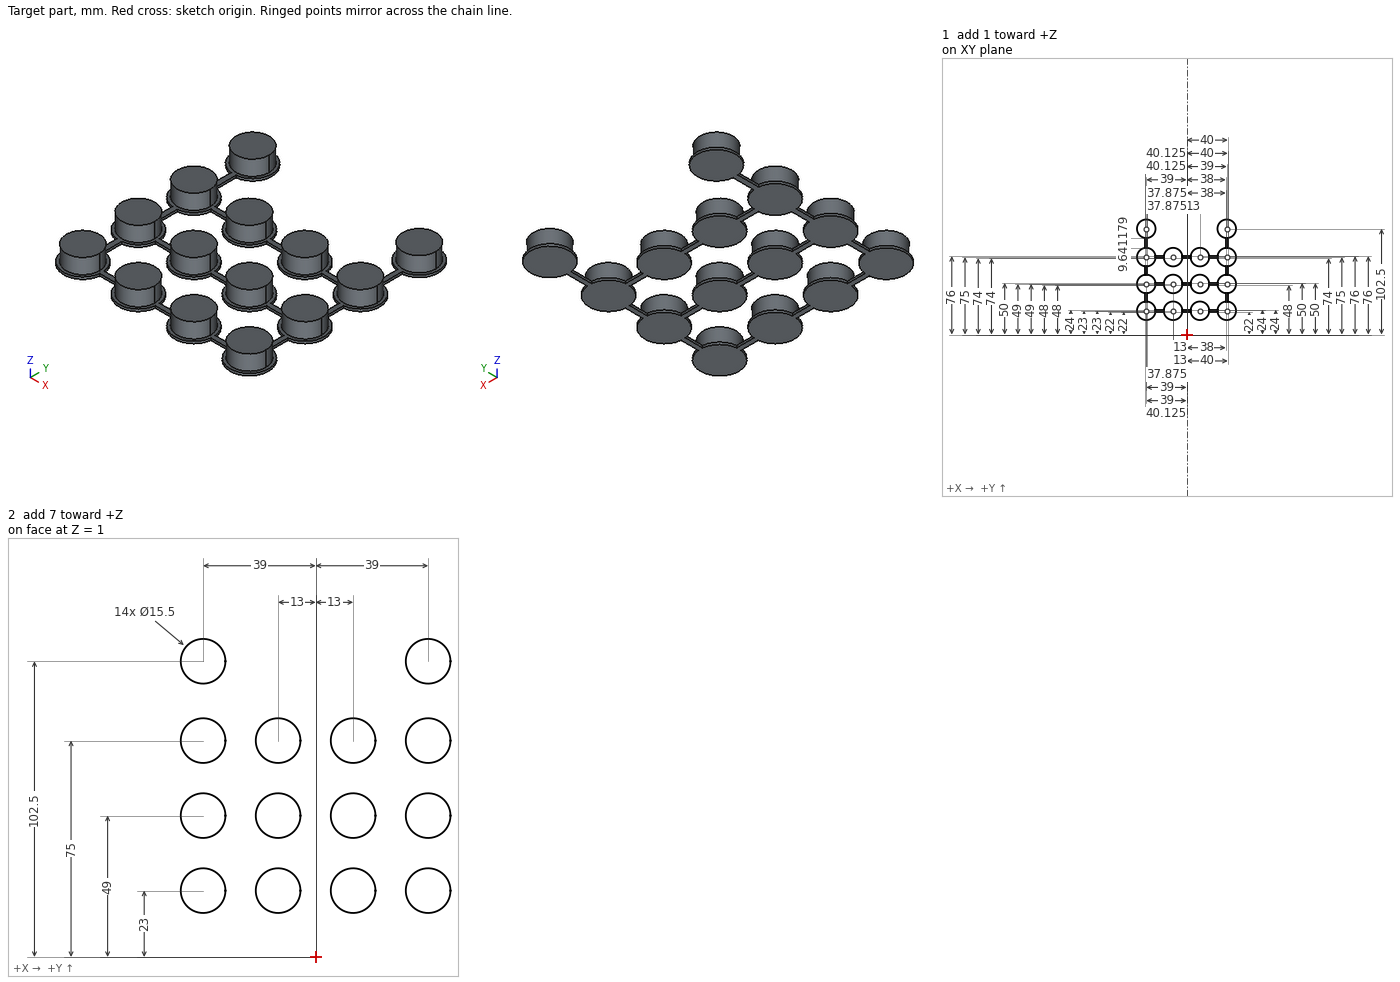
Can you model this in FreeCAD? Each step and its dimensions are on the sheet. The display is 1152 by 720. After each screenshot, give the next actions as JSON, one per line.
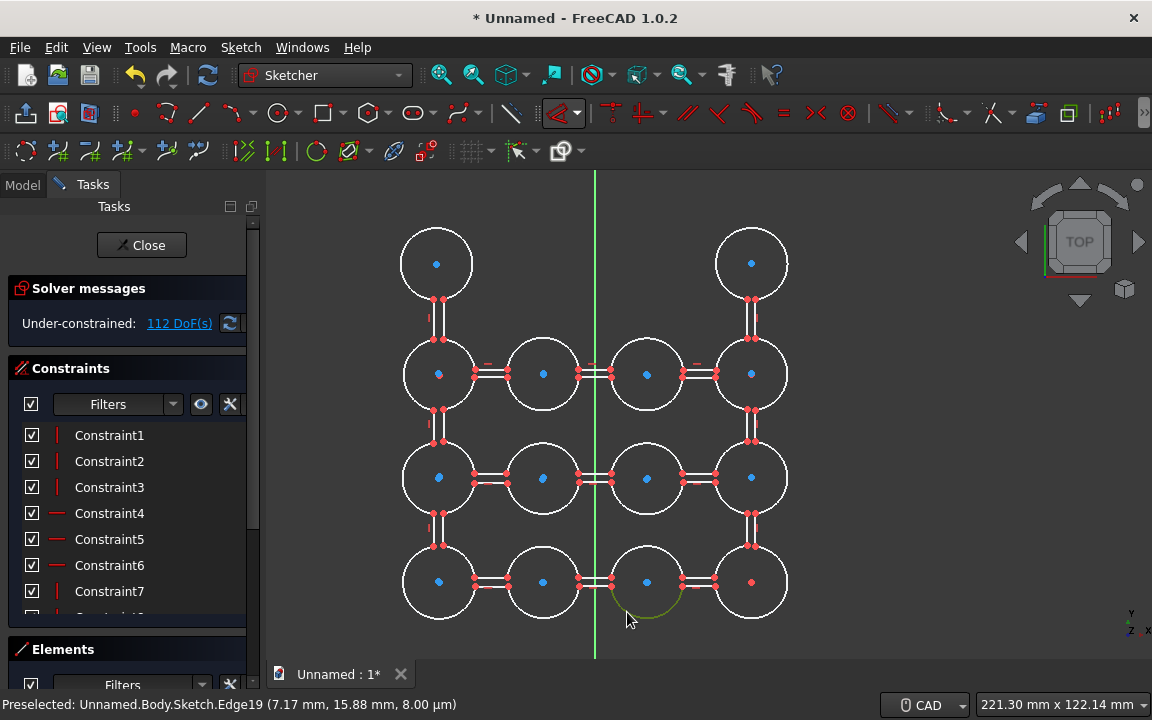
{"action": "left_click", "coordinate": [667, 552]}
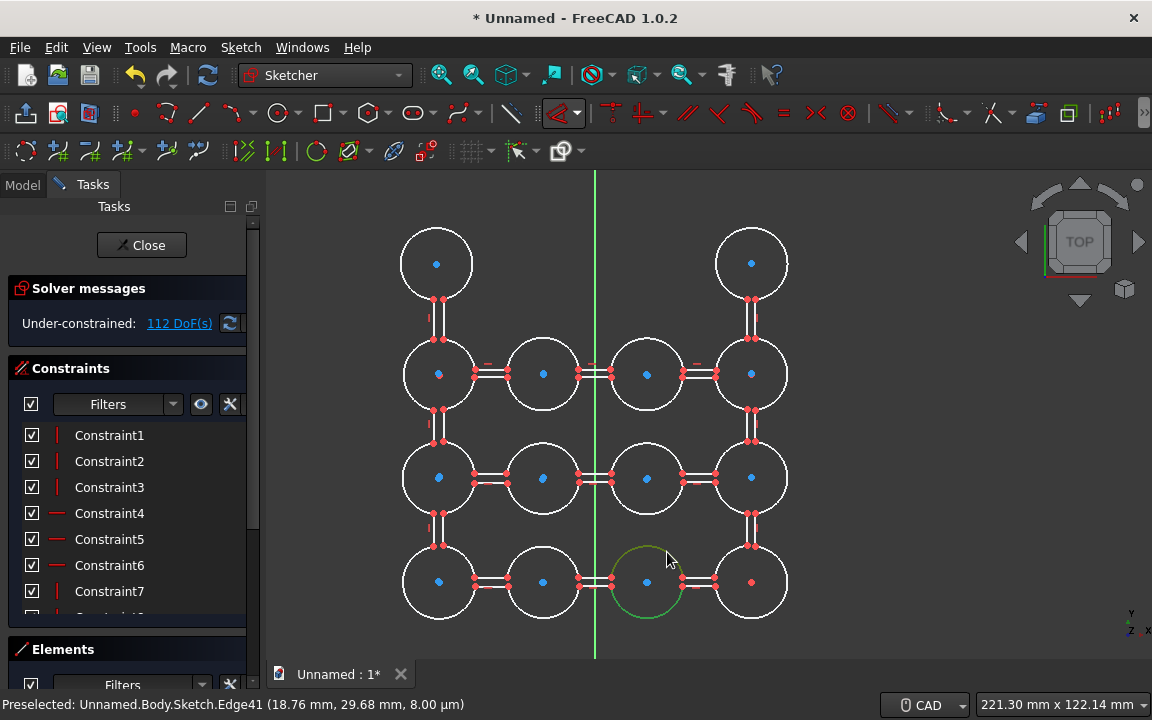
{"action": "left_click", "coordinate": [612, 114]}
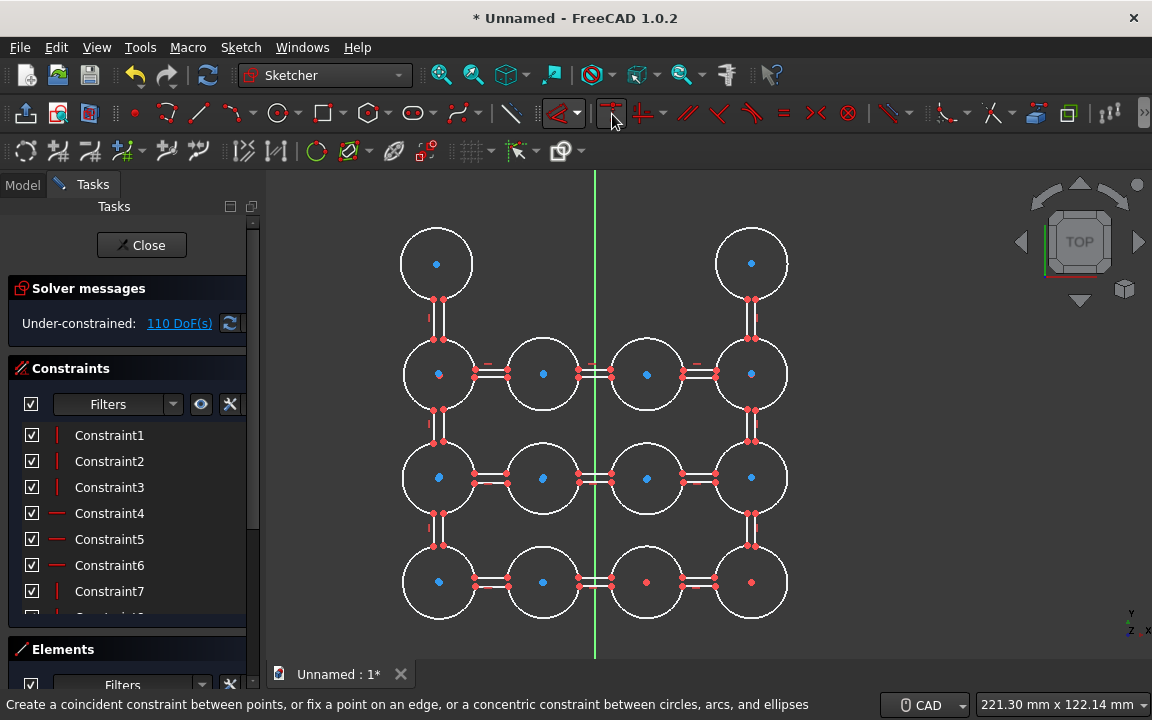
{"action": "left_click", "coordinate": [524, 612]}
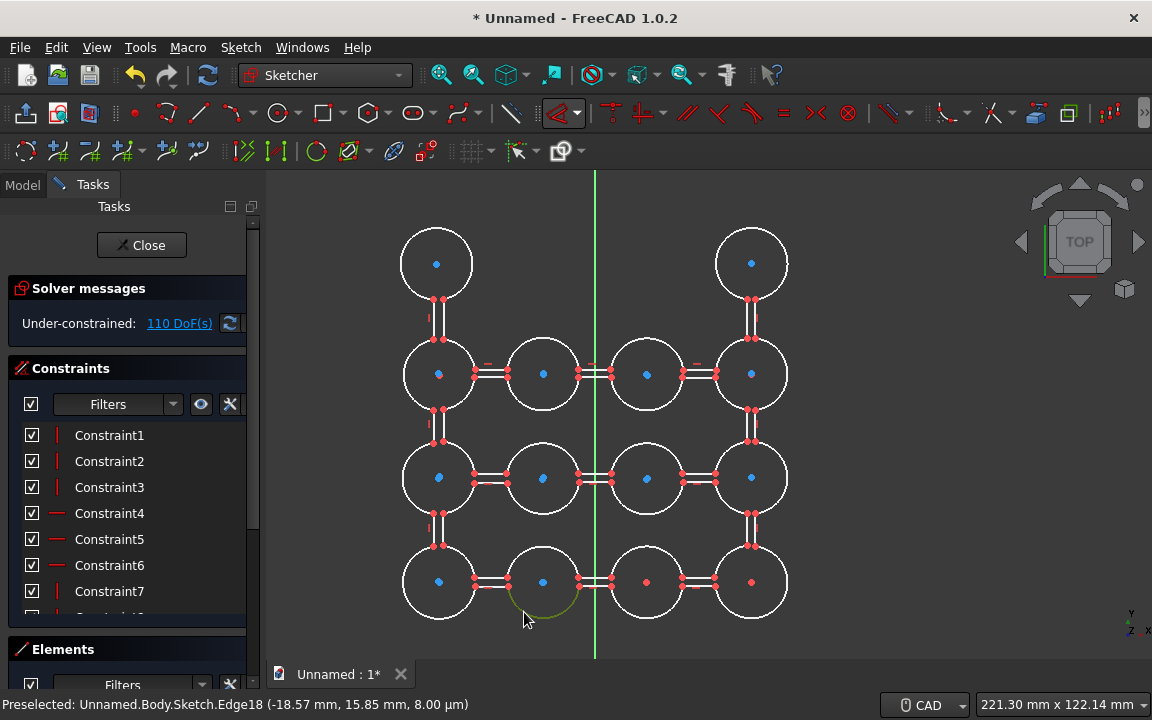
{"action": "left_click", "coordinate": [562, 552]}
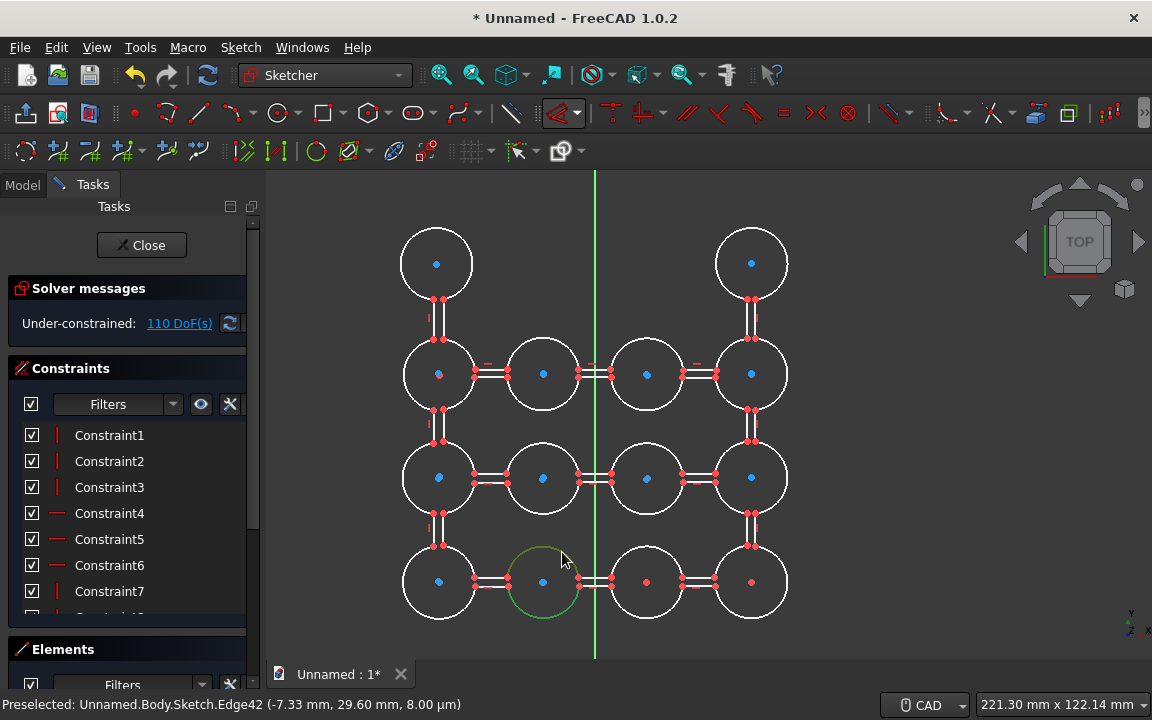
{"action": "left_click", "coordinate": [612, 114]}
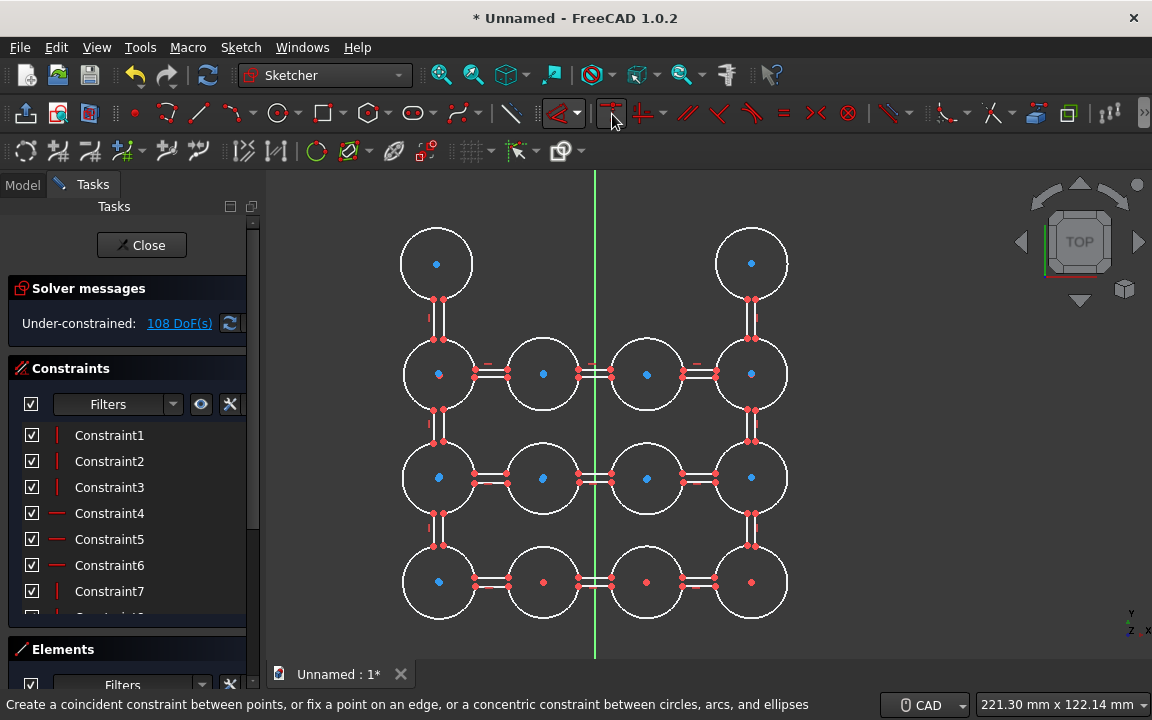
{"action": "left_click", "coordinate": [403, 580]}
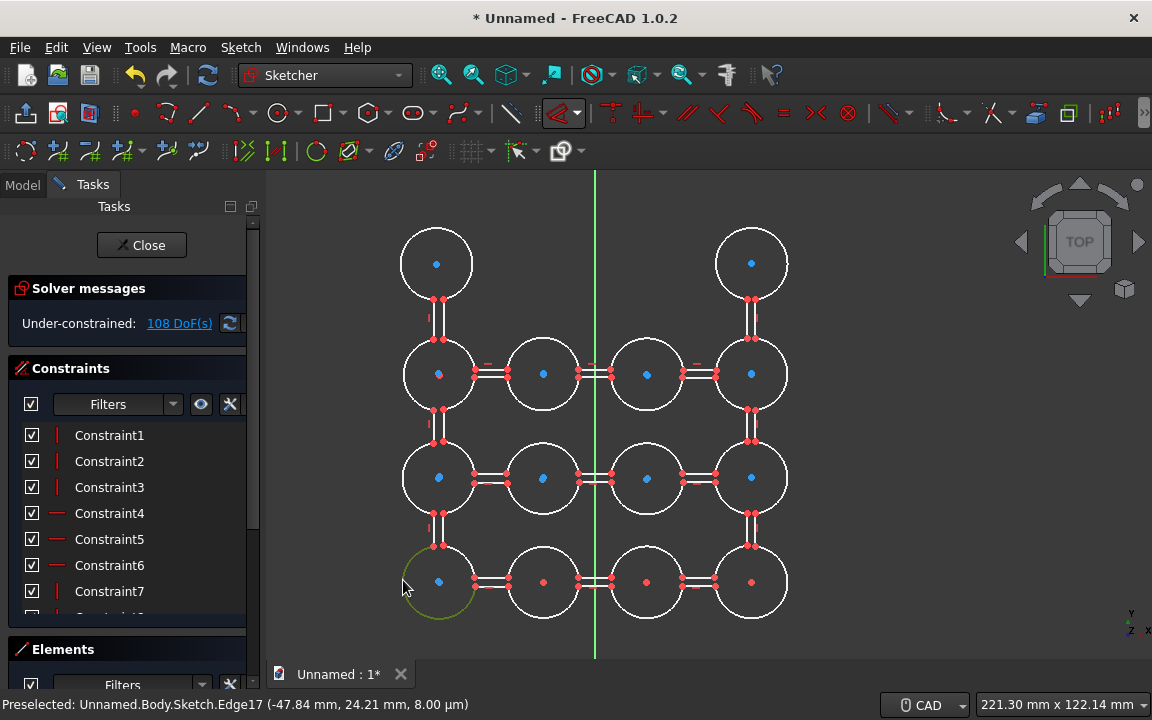
{"action": "left_click", "coordinate": [470, 564]}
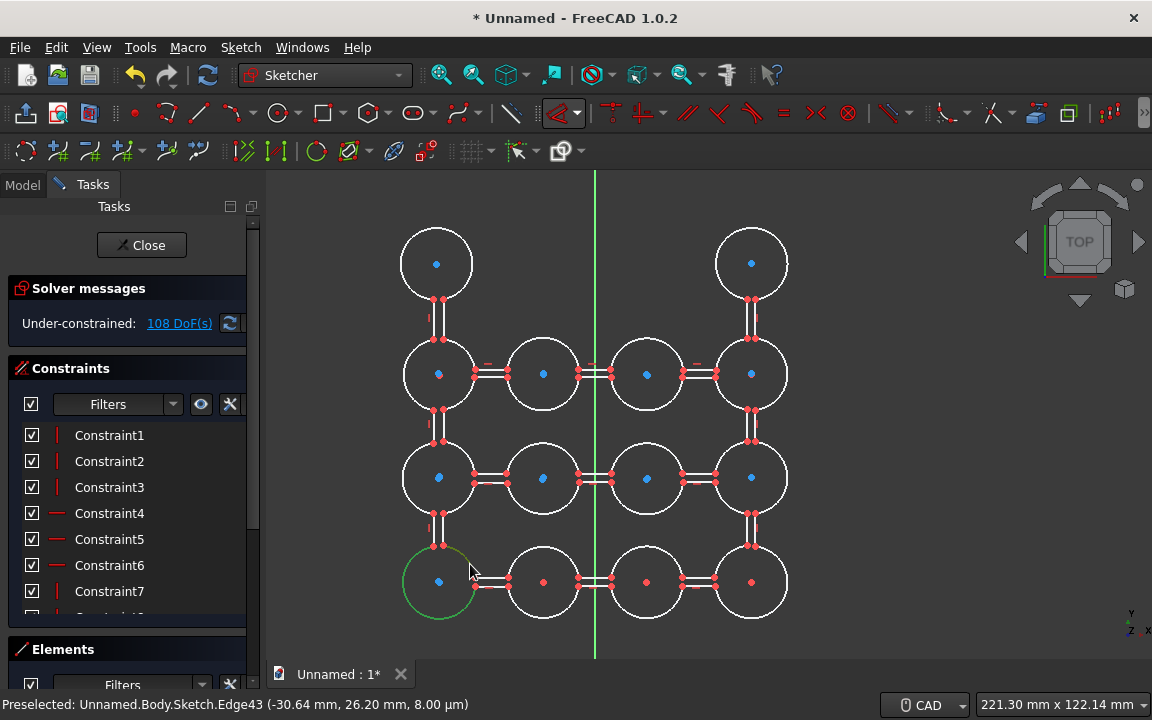
{"action": "left_click", "coordinate": [612, 114]}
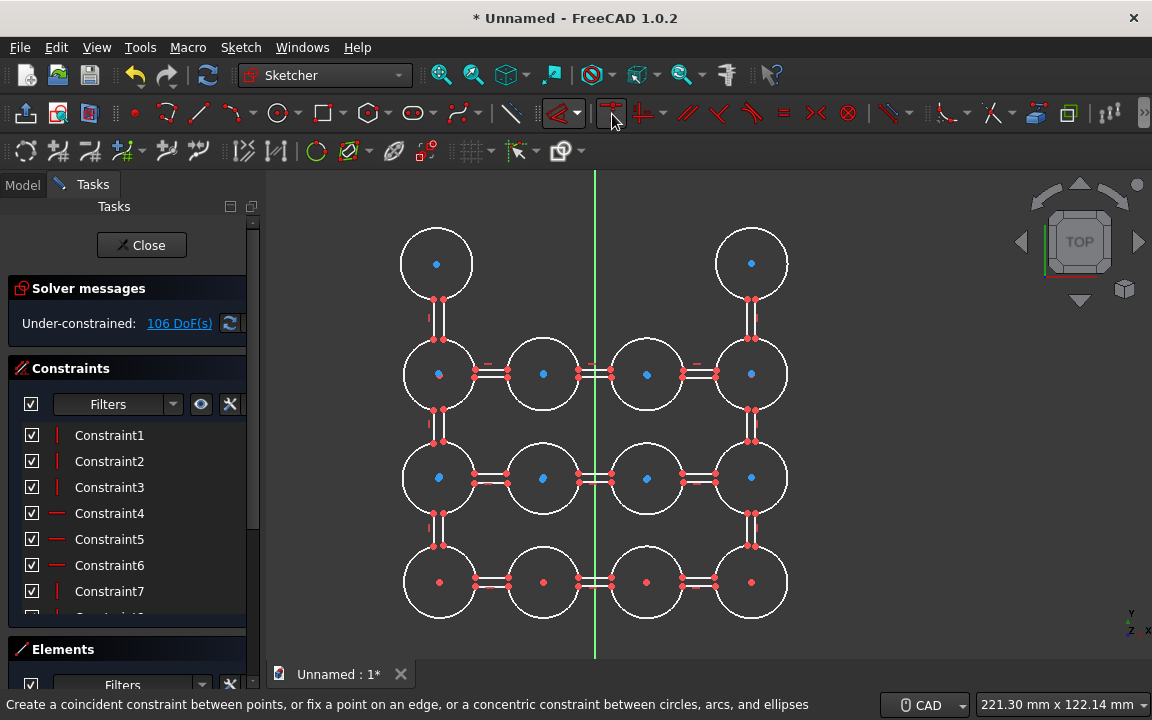
{"action": "left_click", "coordinate": [408, 459]}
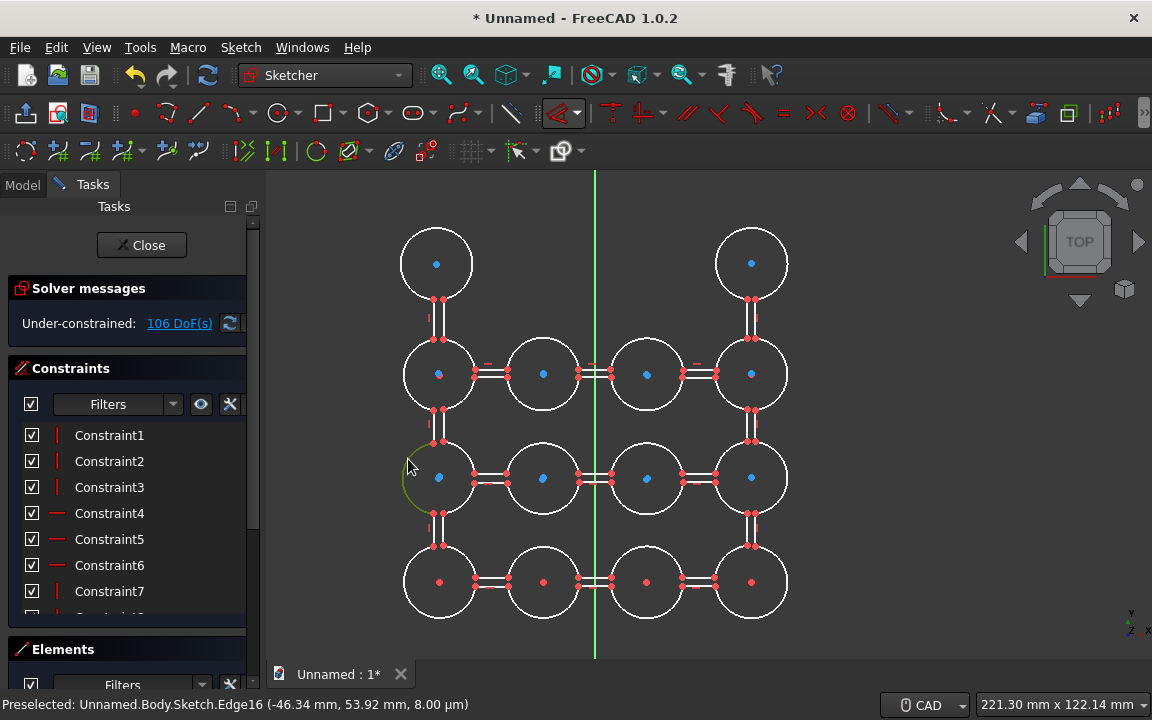
{"action": "left_click", "coordinate": [457, 509]}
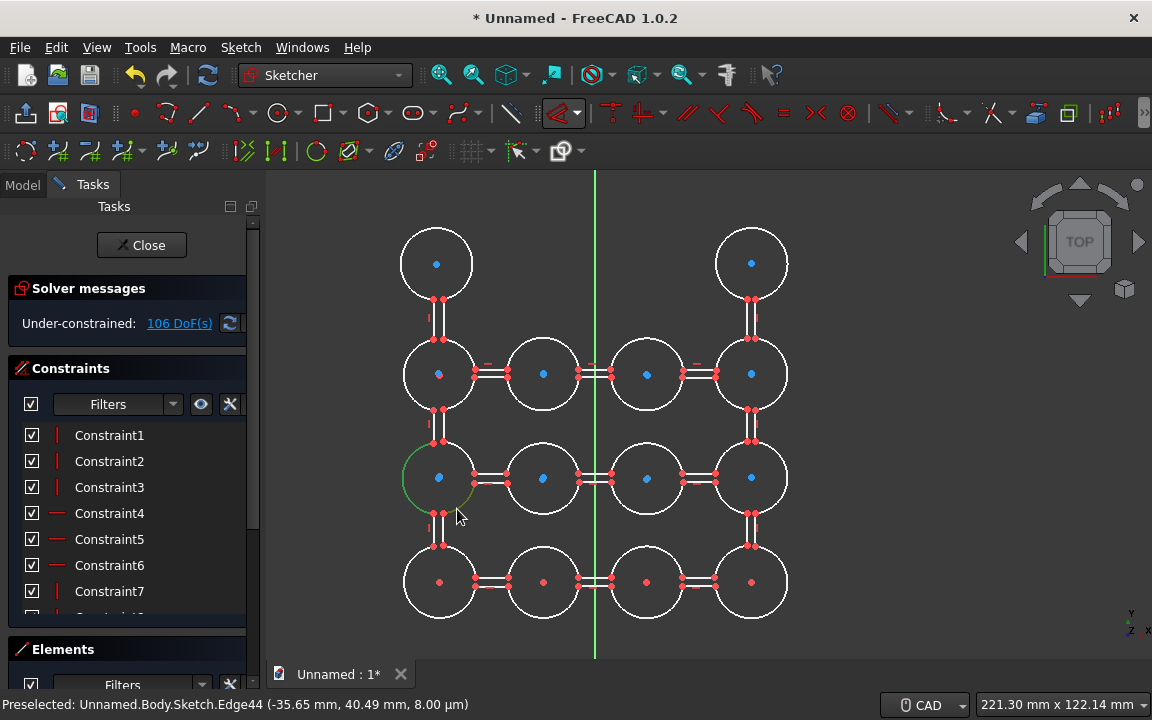
{"action": "left_click", "coordinate": [612, 114]}